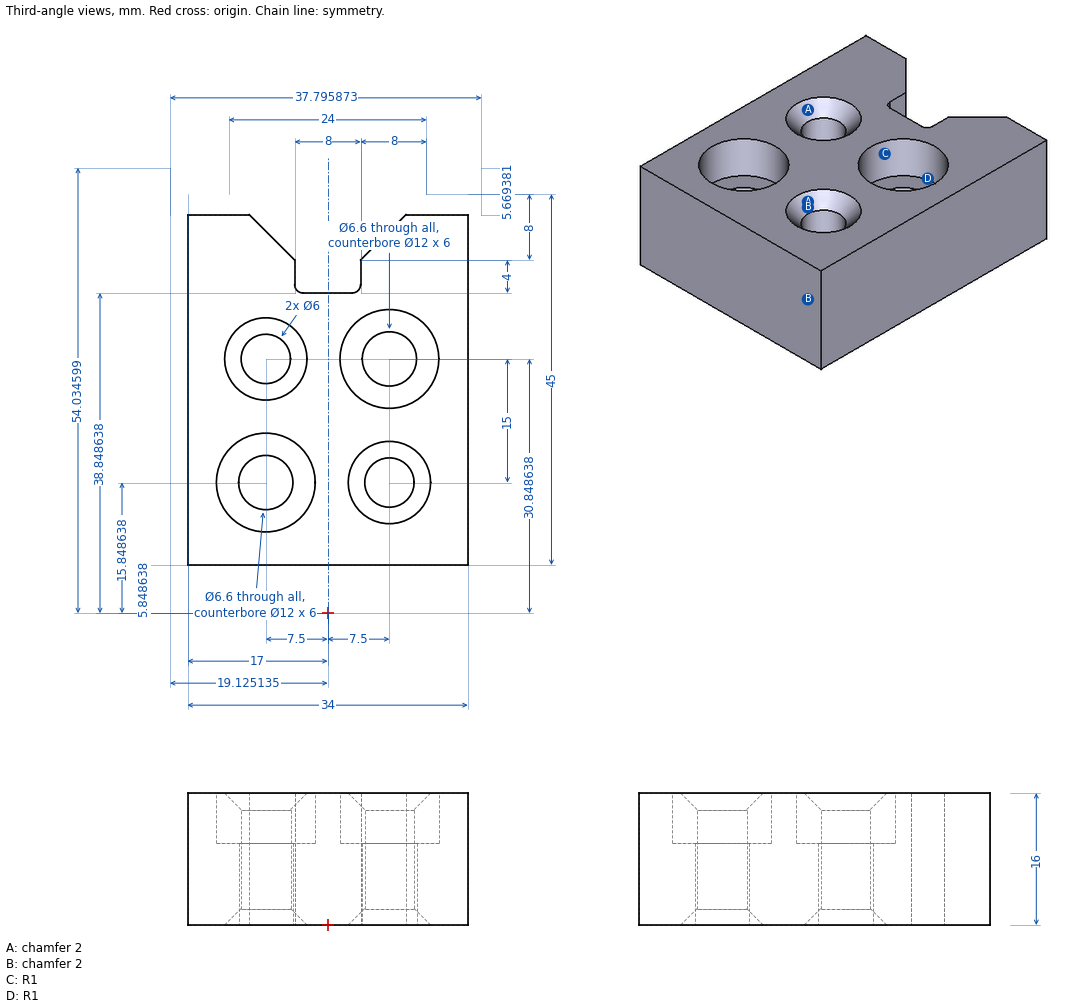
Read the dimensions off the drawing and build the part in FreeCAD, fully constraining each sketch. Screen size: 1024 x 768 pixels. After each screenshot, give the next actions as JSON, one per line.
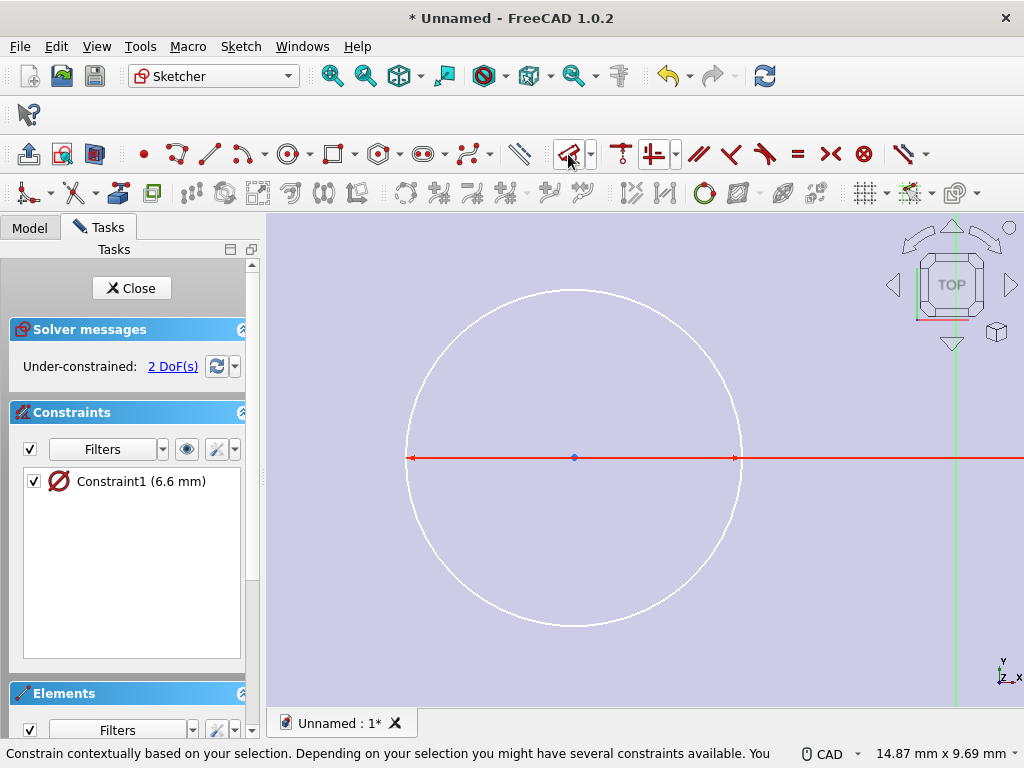
{"action": "left_click", "coordinate": [574, 458]}
{"action": "left_click", "coordinate": [717, 424]}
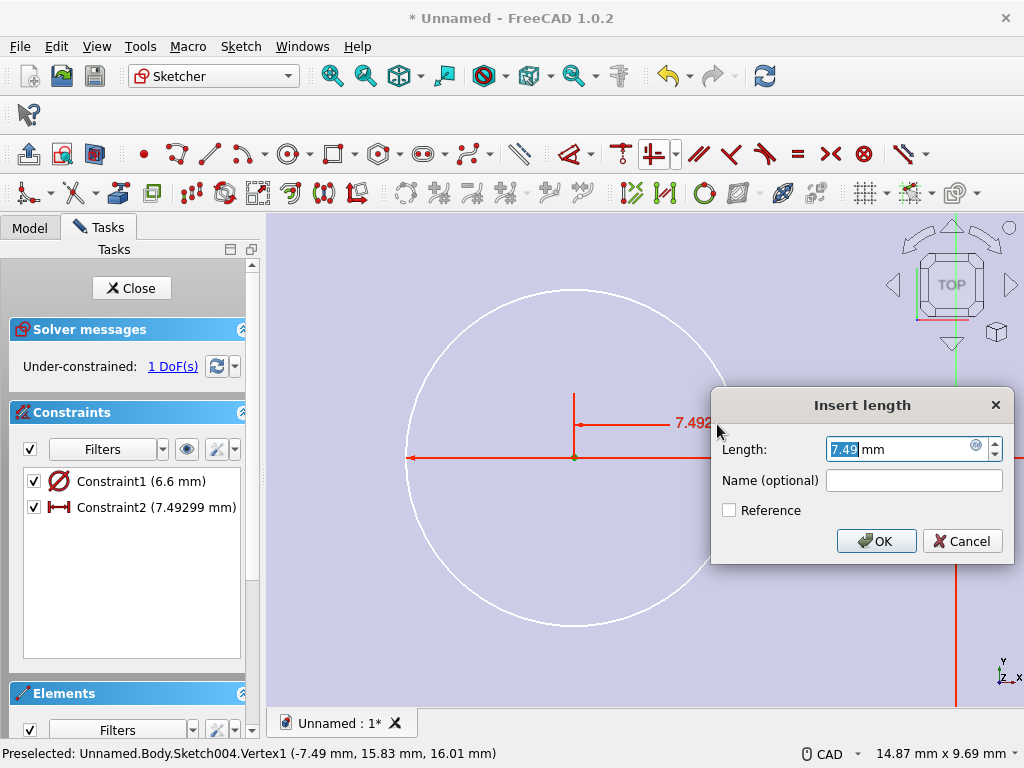
{"action": "type", "text": "7.5"}
{"action": "key", "text": "Return"}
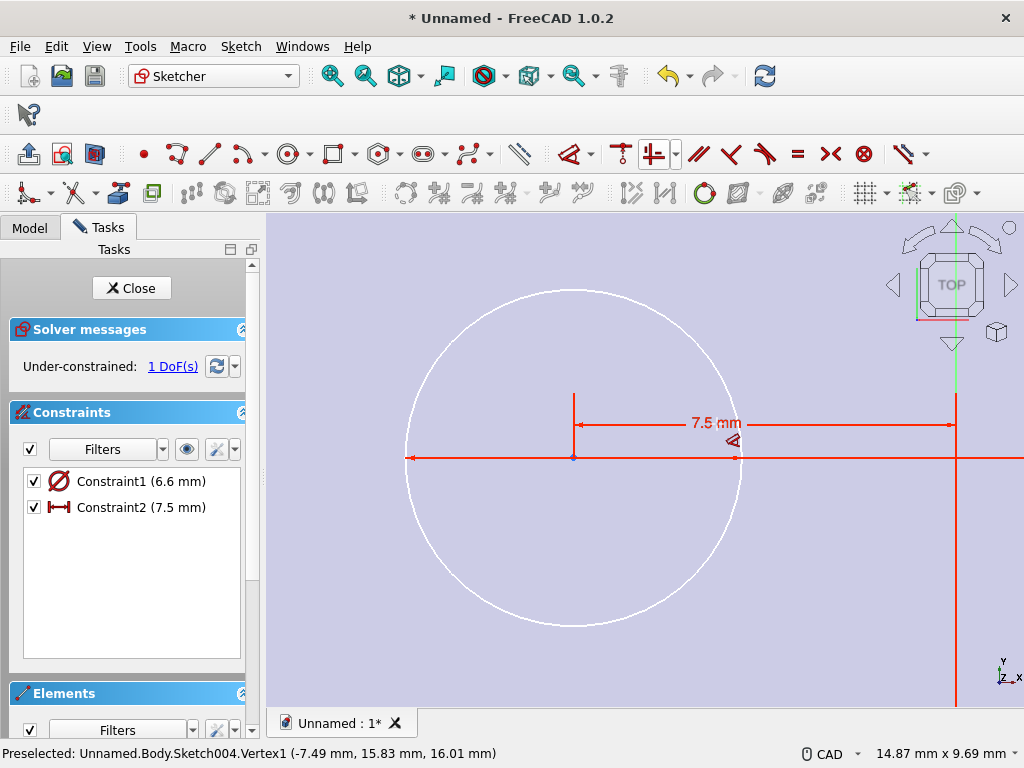
{"action": "left_click", "coordinate": [574, 458]}
{"action": "left_click", "coordinate": [540, 569]}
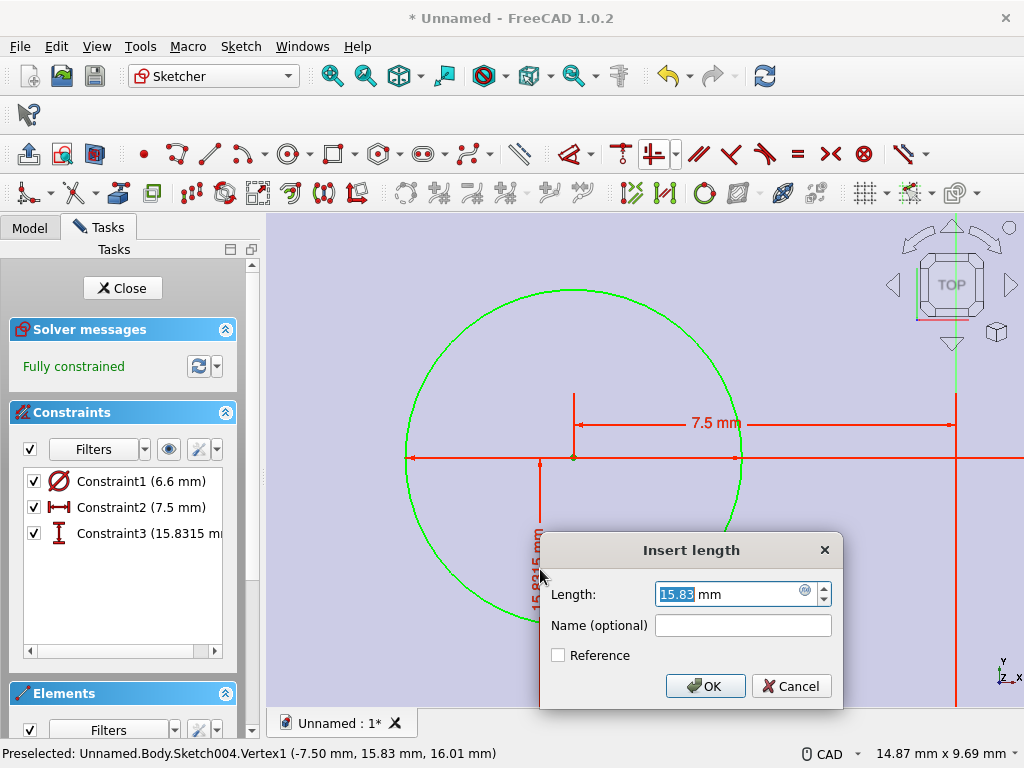
{"action": "type", "text": "15.848638"}
{"action": "key", "text": "Return"}
{"action": "key", "text": "Escape"}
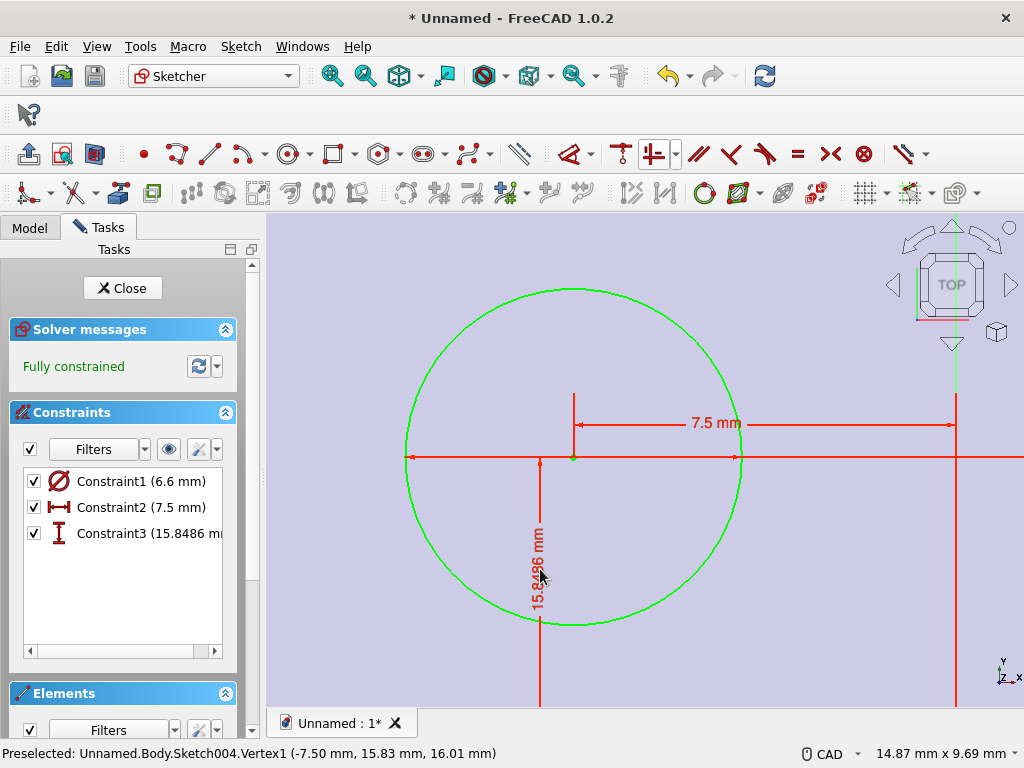
{"action": "left_click", "coordinate": [123, 288]}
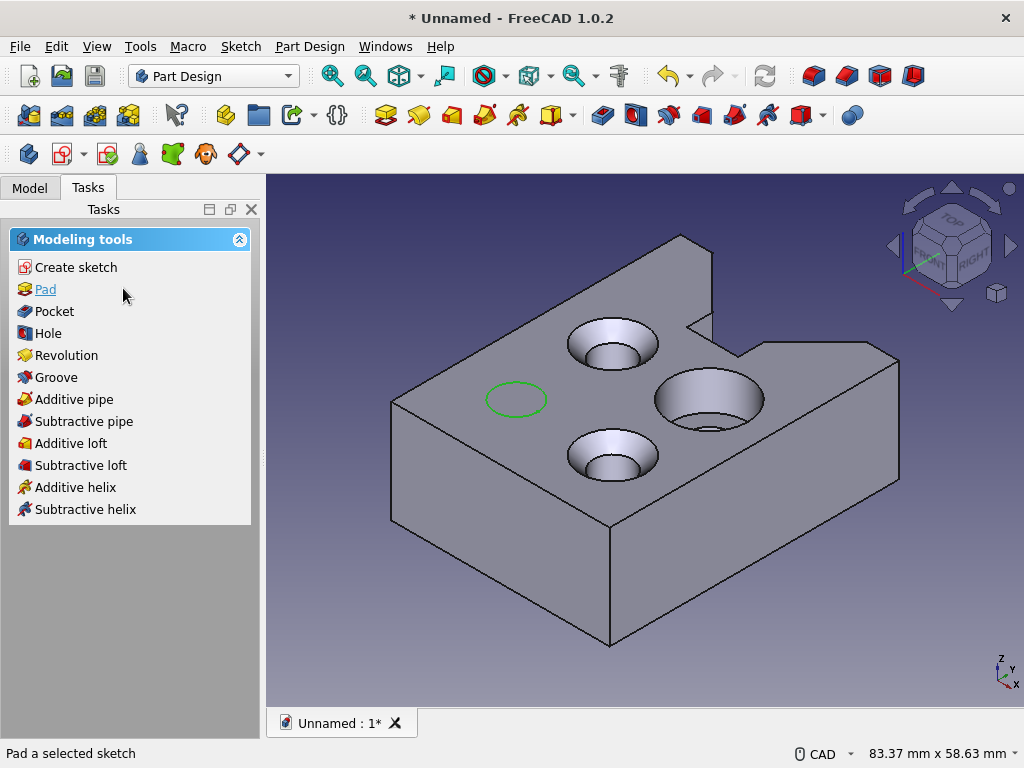
{"action": "left_click", "coordinate": [636, 116]}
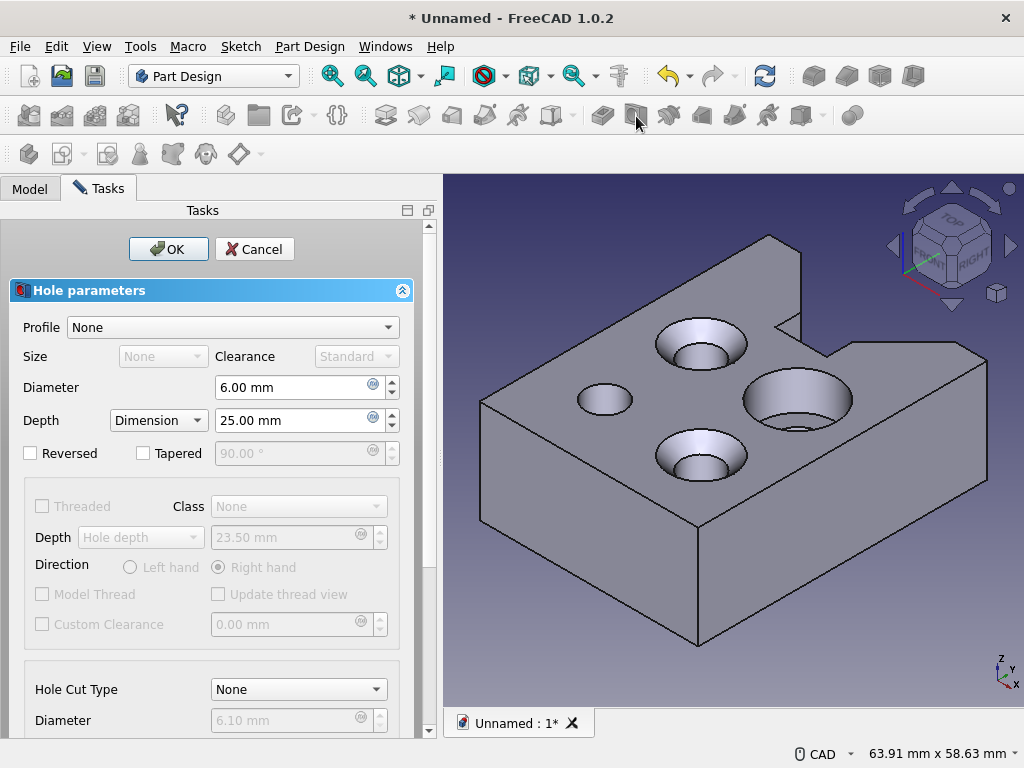
{"action": "triple_click", "coordinate": [300, 388]}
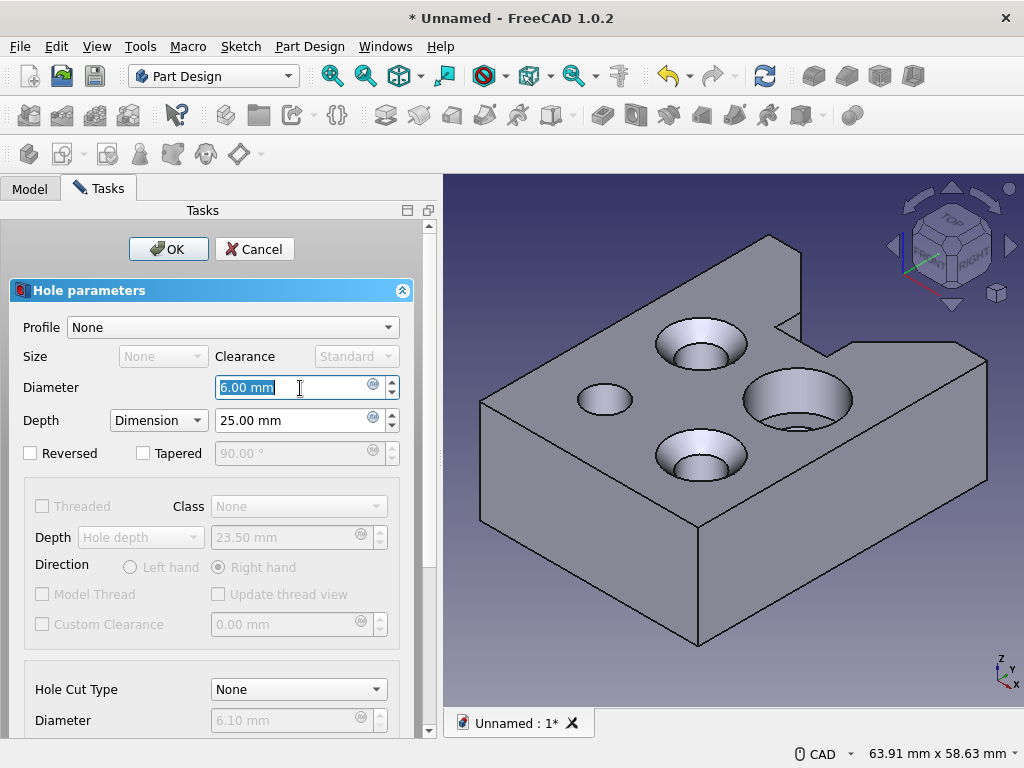
{"action": "type", "text": "6.6"}
{"action": "key", "text": "Tab"}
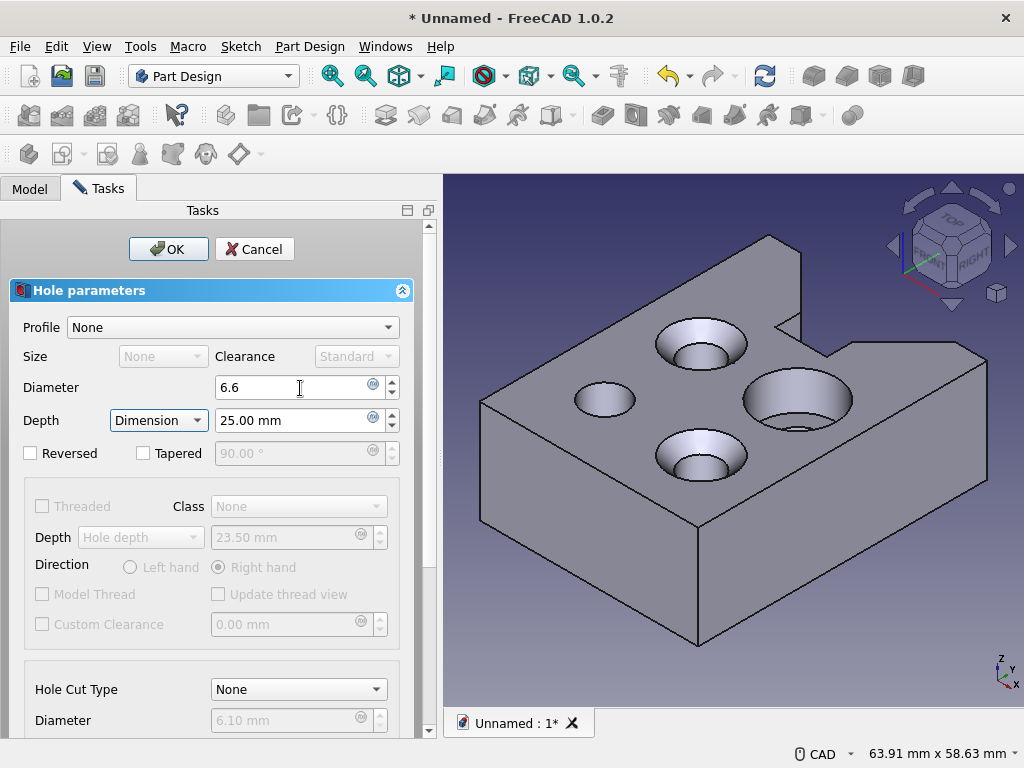
{"action": "left_click", "coordinate": [160, 420]}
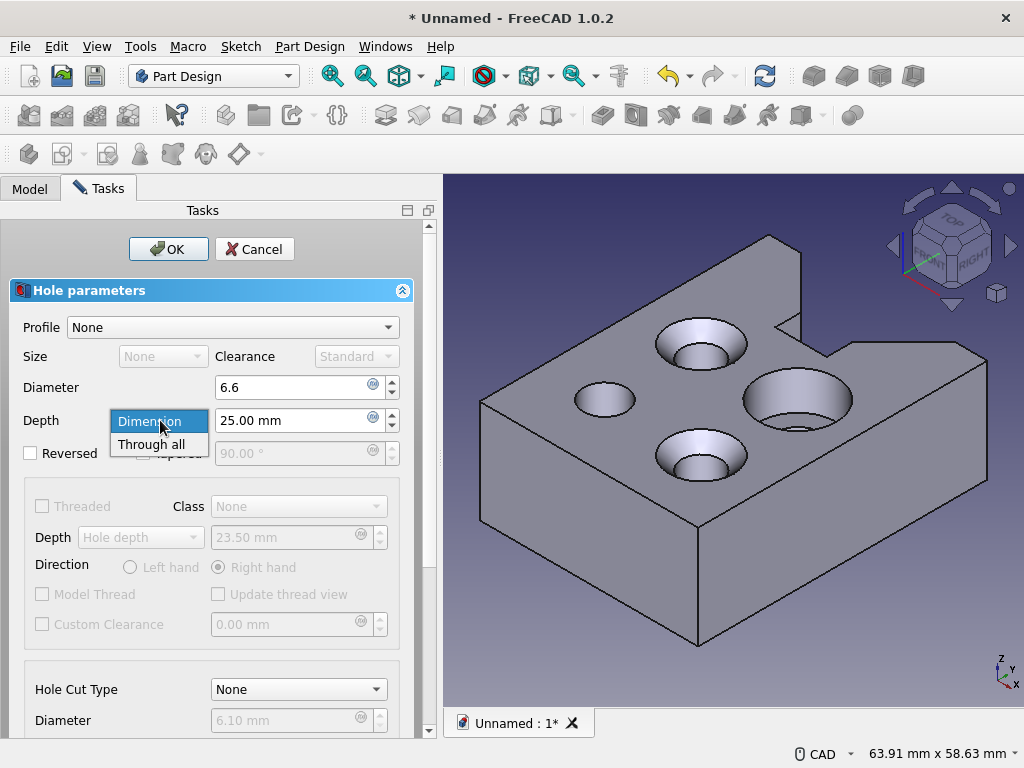
{"action": "left_click", "coordinate": [158, 444]}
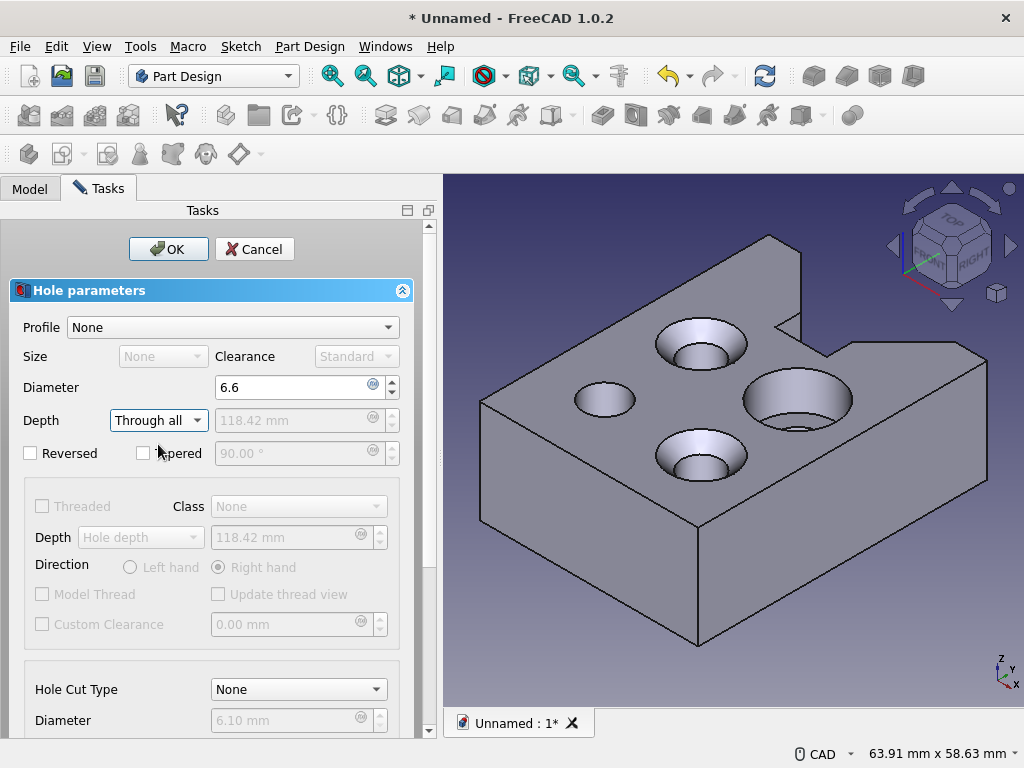
{"action": "left_click", "coordinate": [300, 690]}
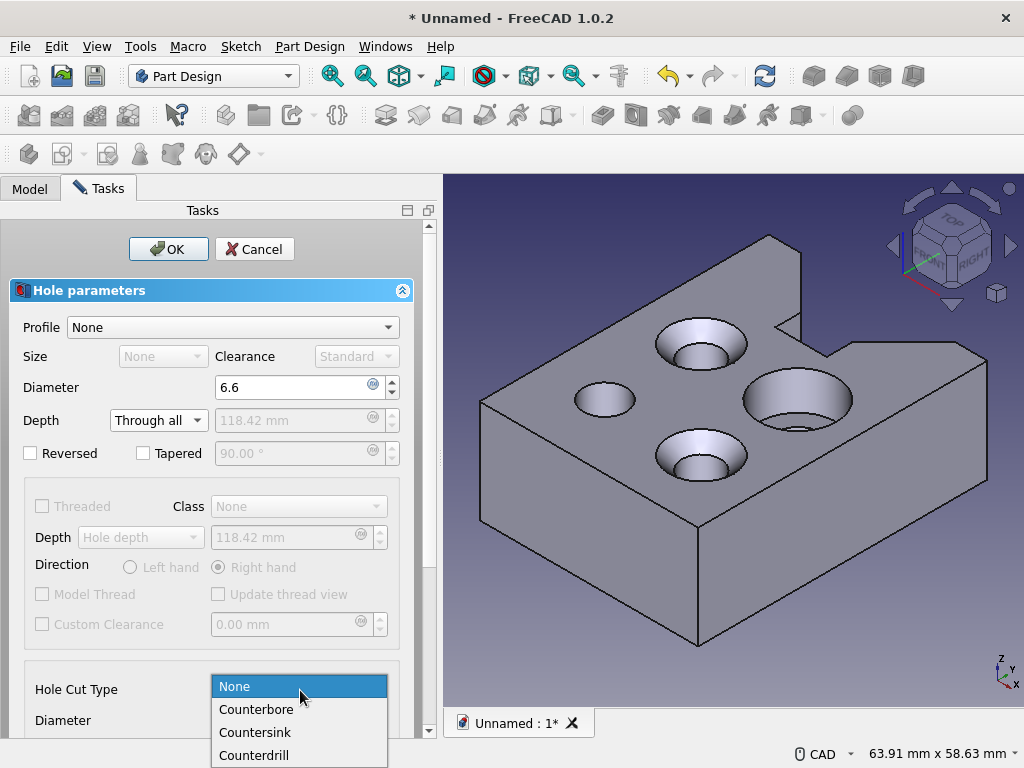
{"action": "left_click", "coordinate": [298, 710]}